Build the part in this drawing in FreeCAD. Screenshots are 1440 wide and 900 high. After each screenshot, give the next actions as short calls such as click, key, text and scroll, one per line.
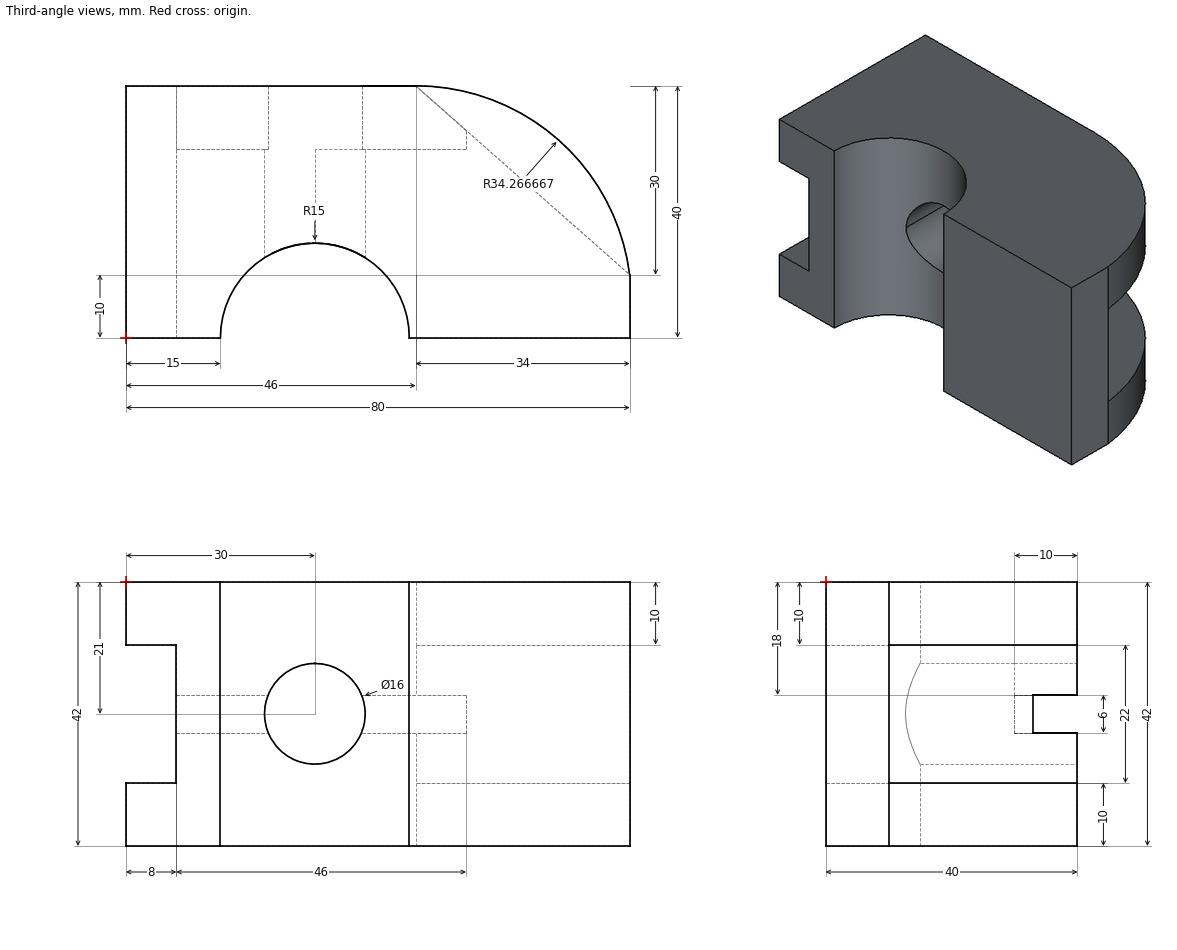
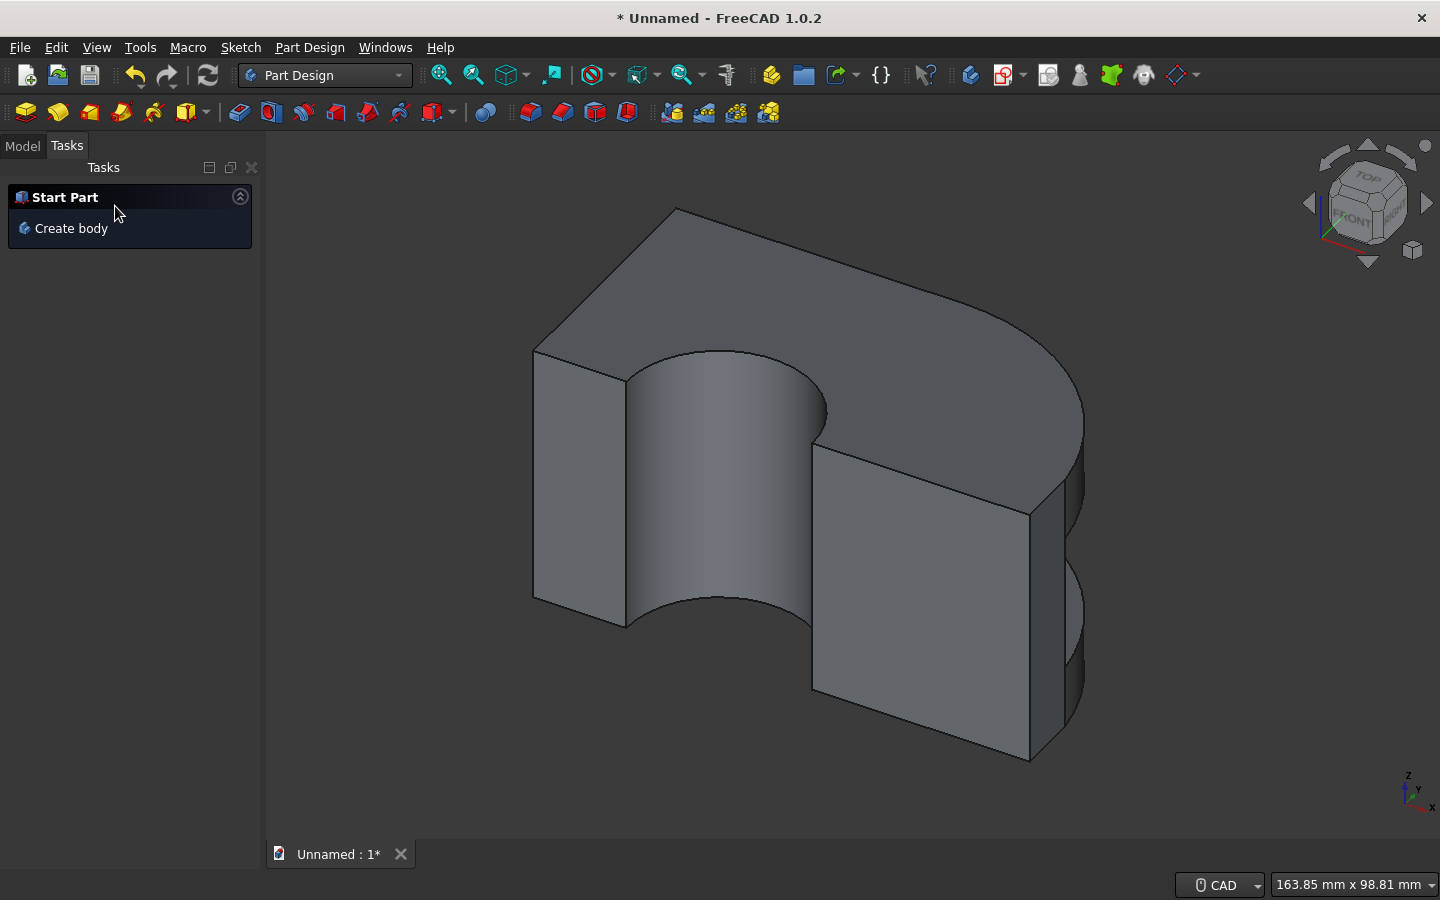
key(4)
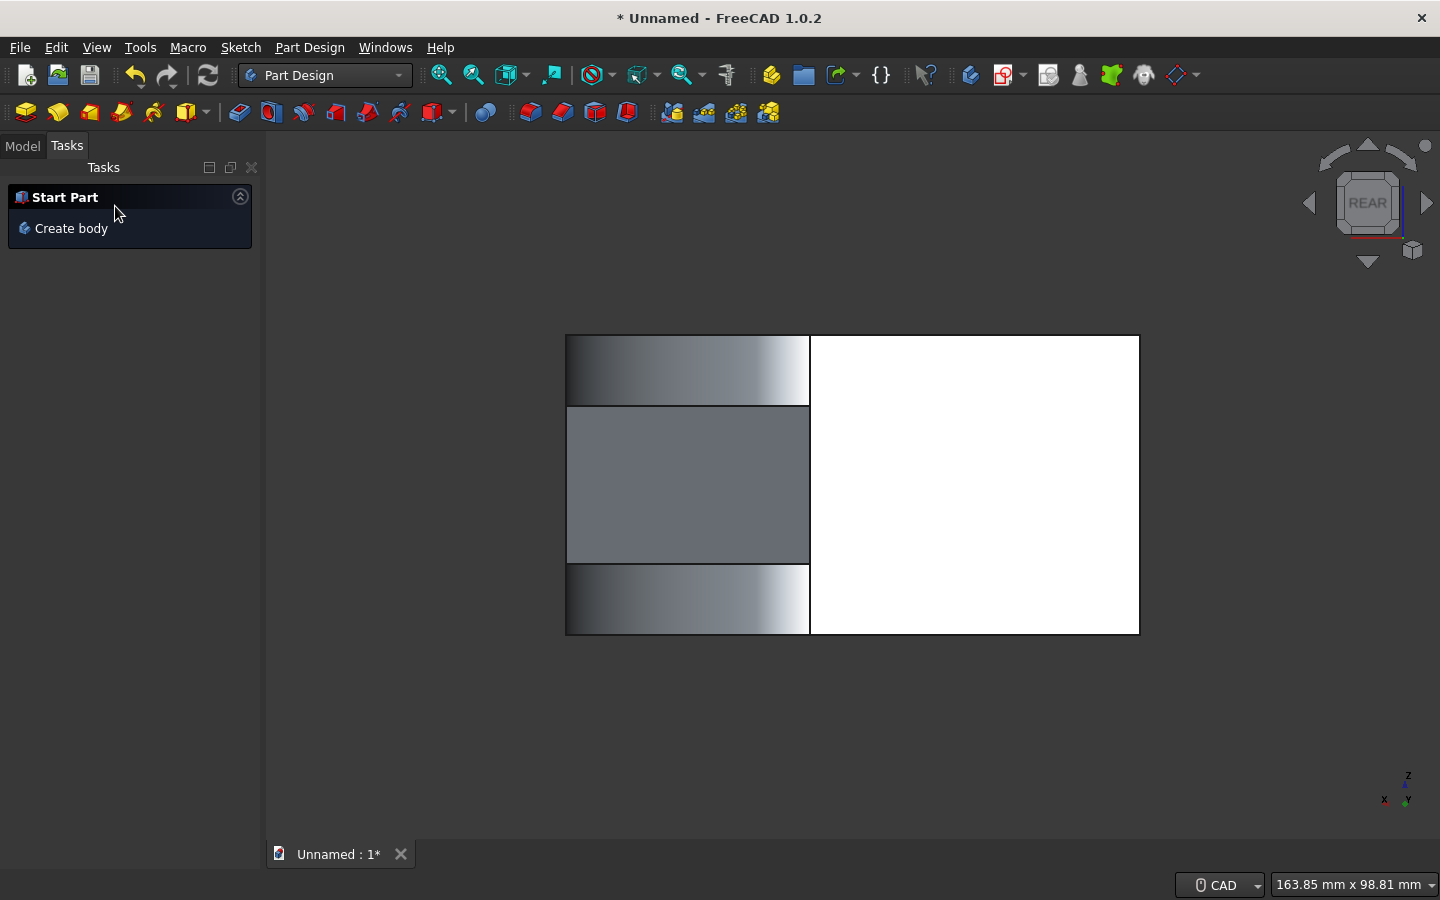
click(975, 484)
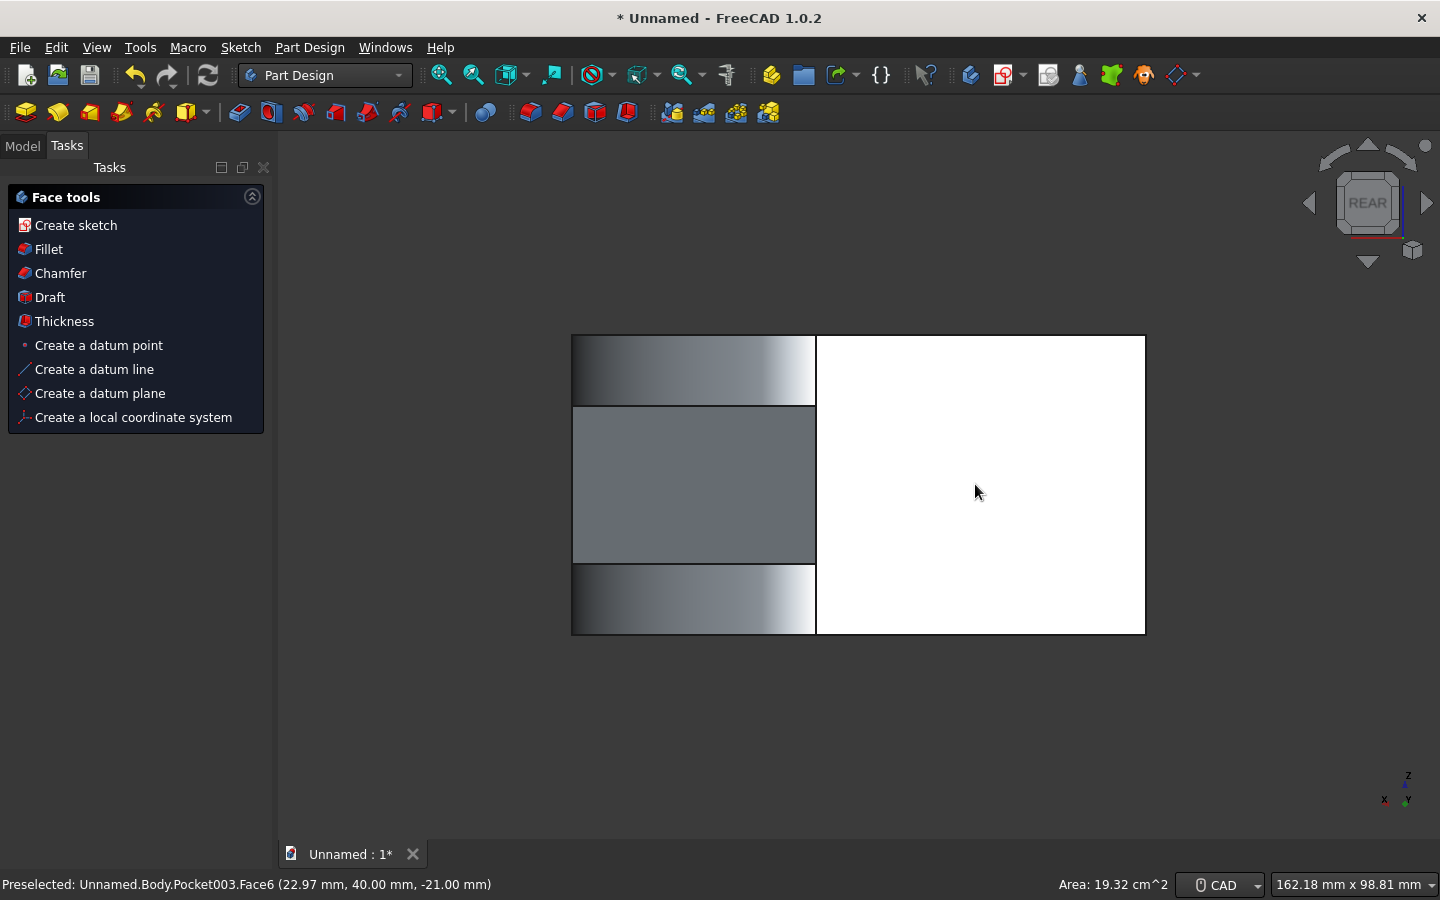
click(1004, 76)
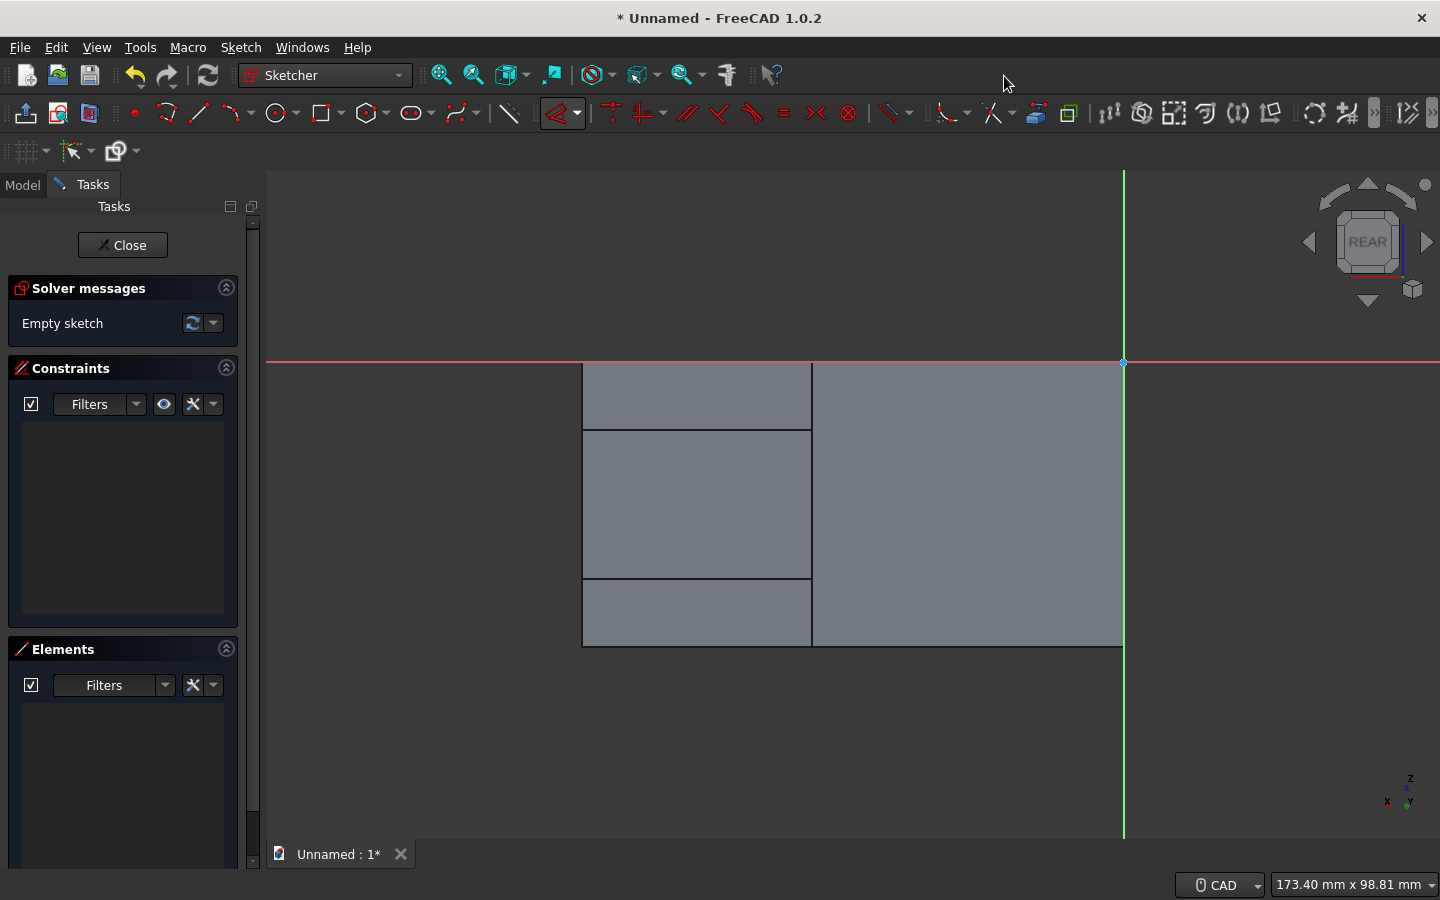
scroll(1167, 425, up, 4)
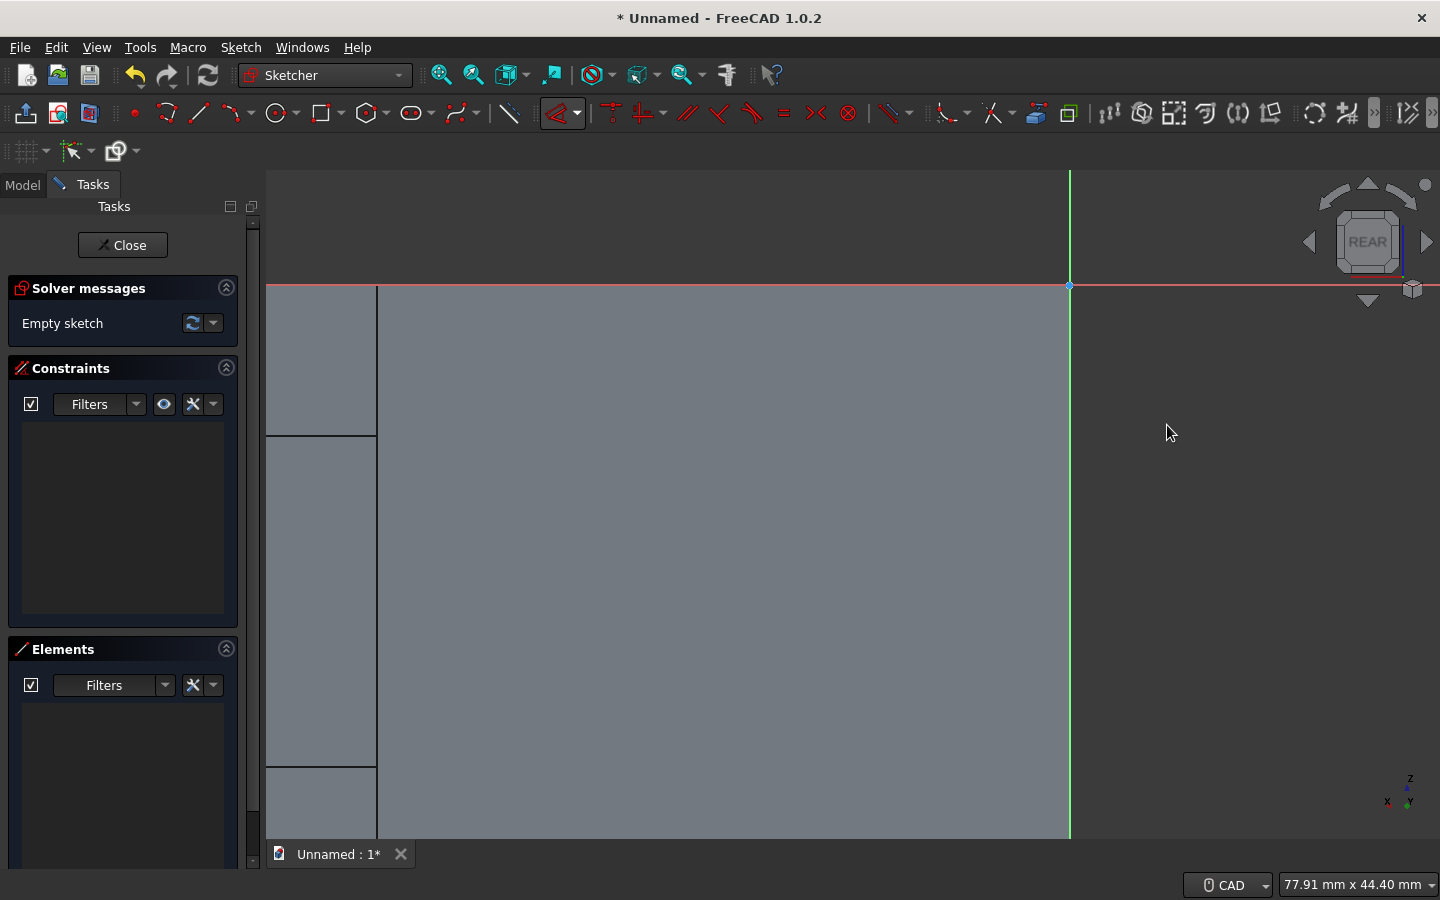
click(276, 114)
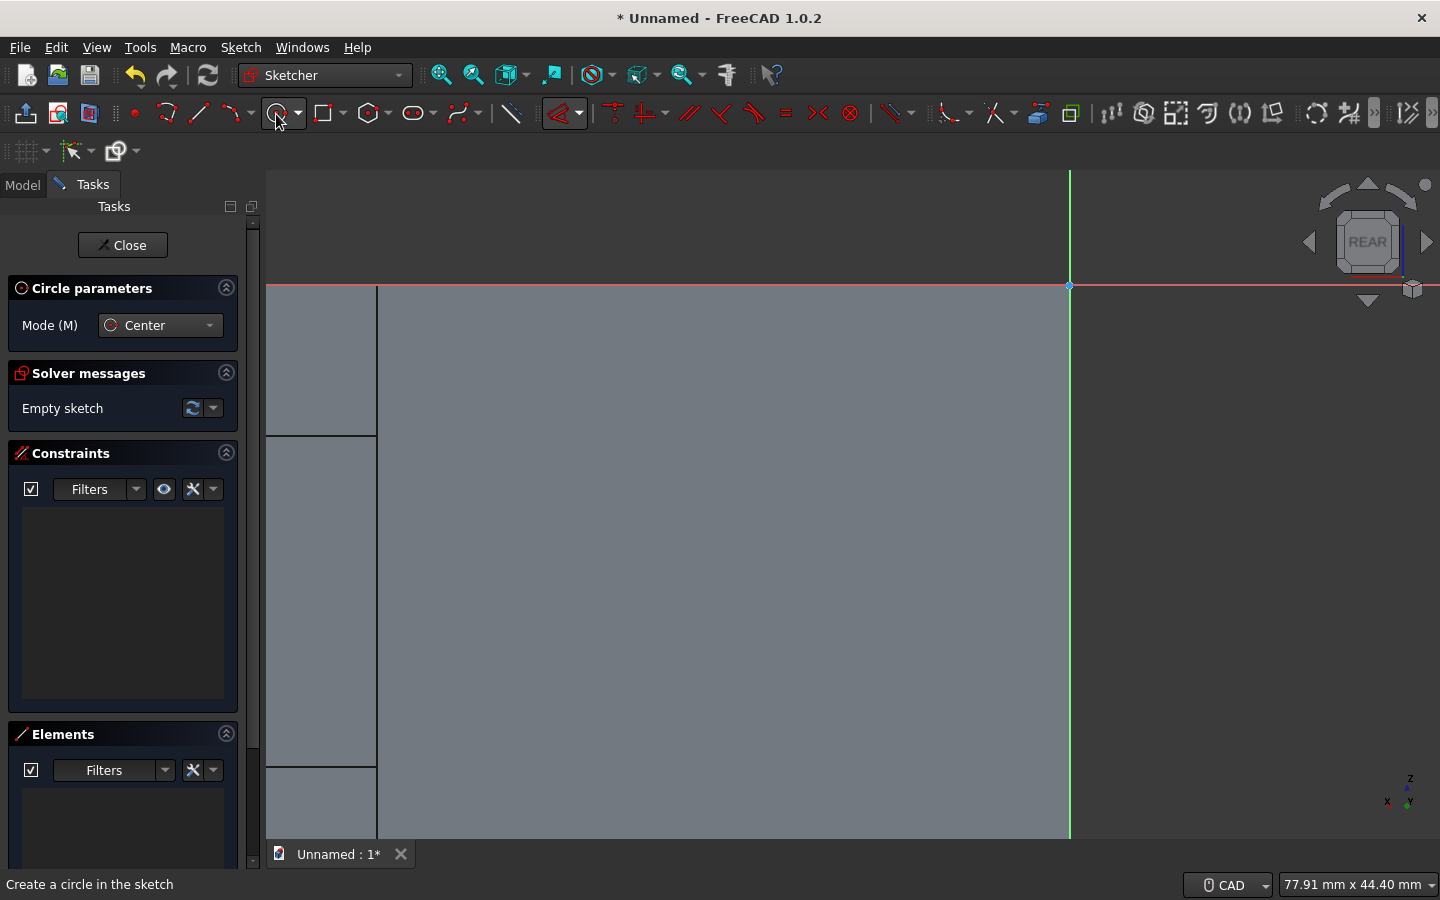
click(618, 601)
move(703, 516)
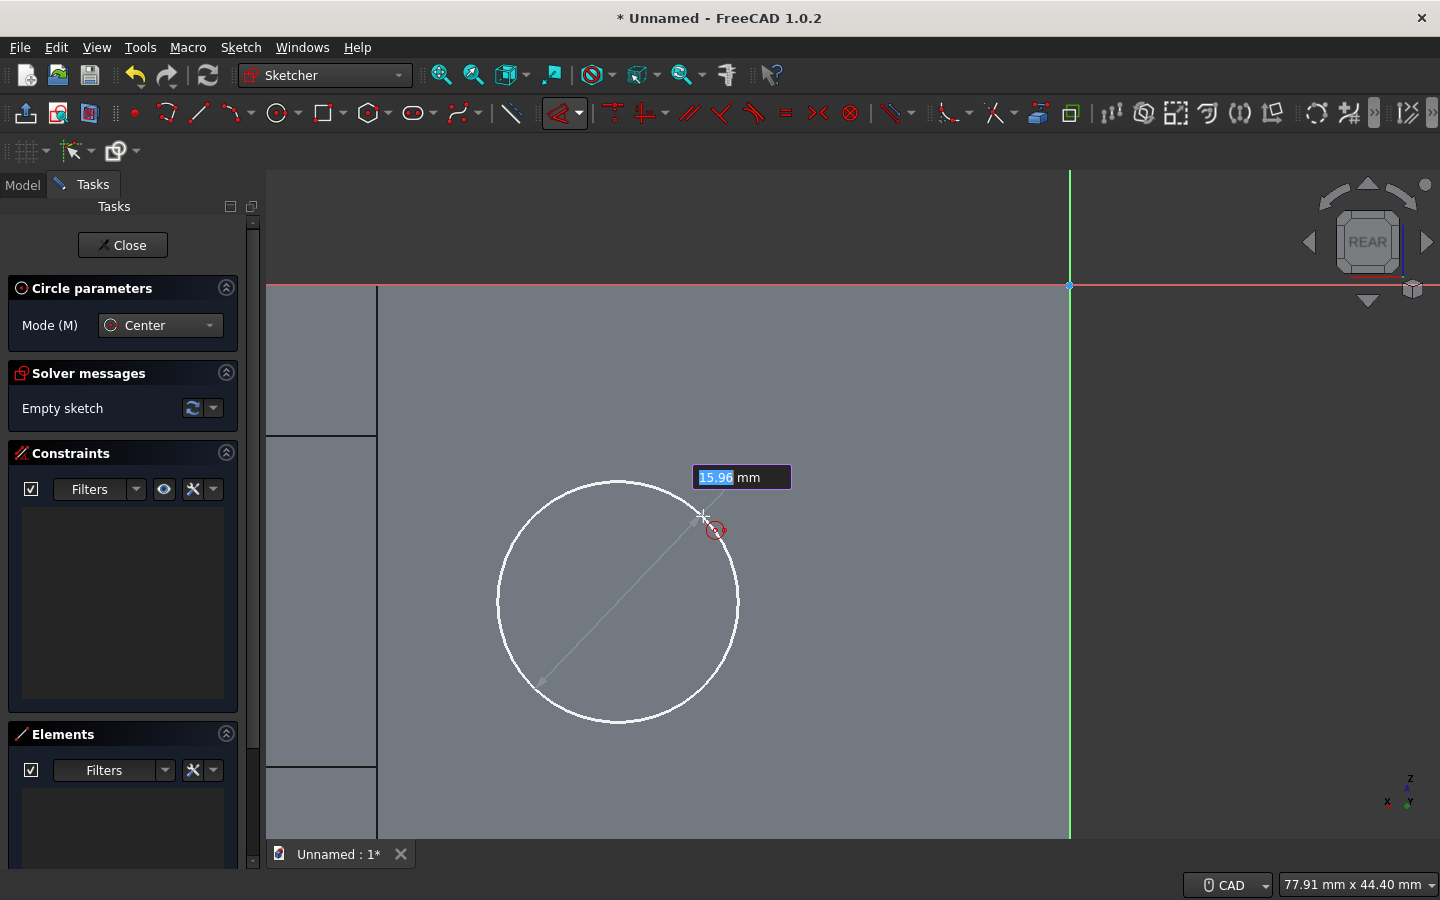
text(16)
key(Return)
key(Escape)